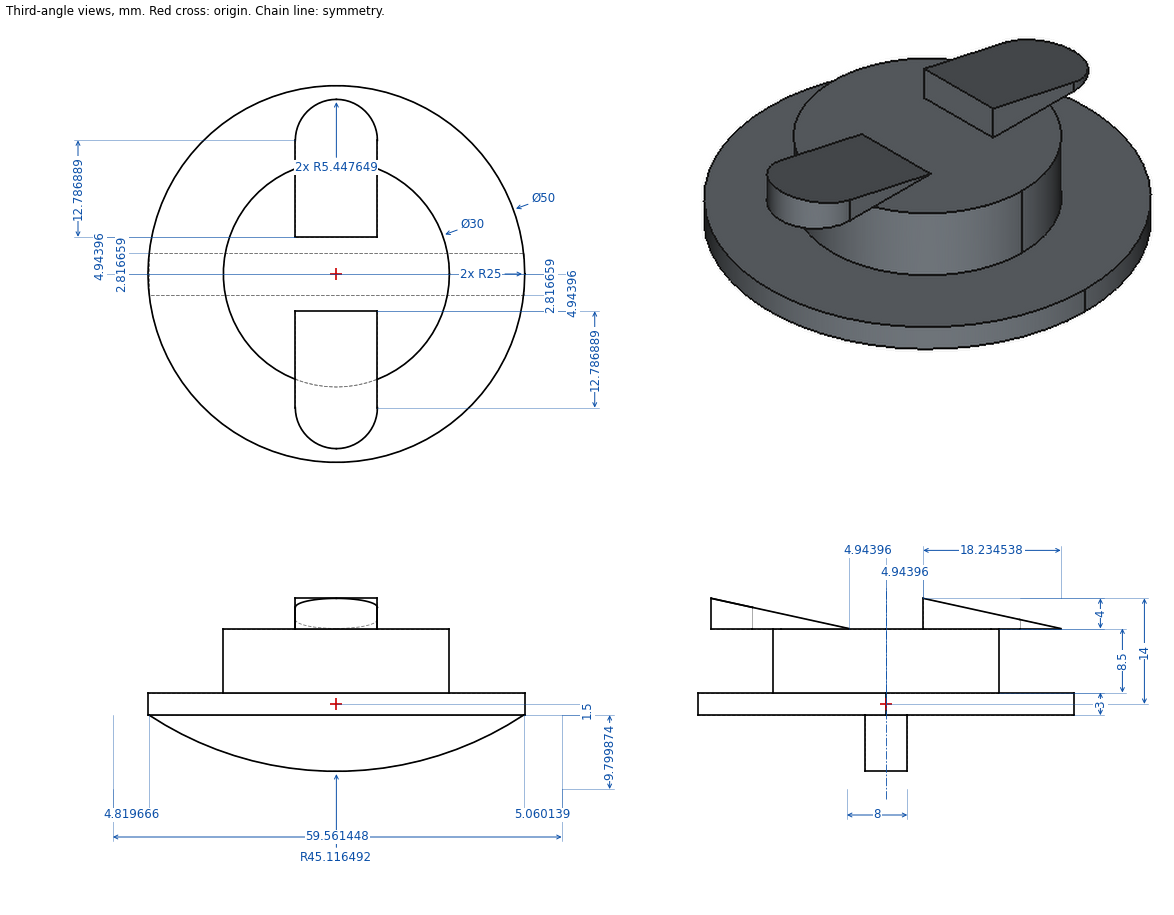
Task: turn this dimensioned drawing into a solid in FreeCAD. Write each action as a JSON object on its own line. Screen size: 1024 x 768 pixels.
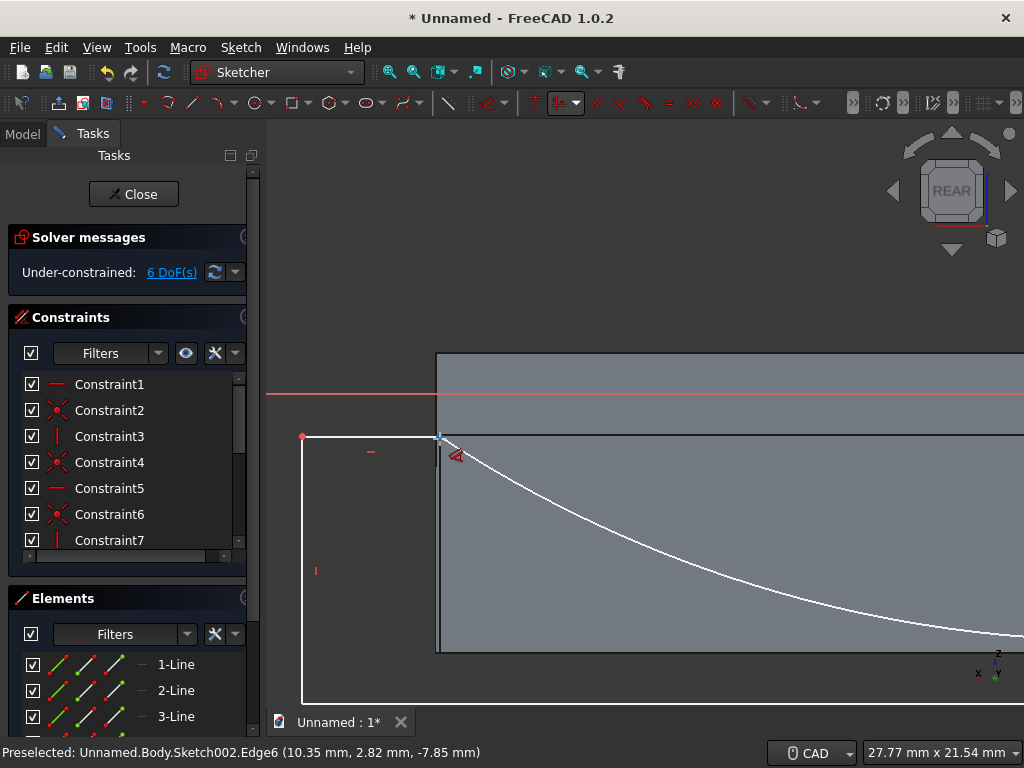
{"action": "left_click", "coordinate": [440, 437]}
{"action": "left_click", "coordinate": [406, 415]}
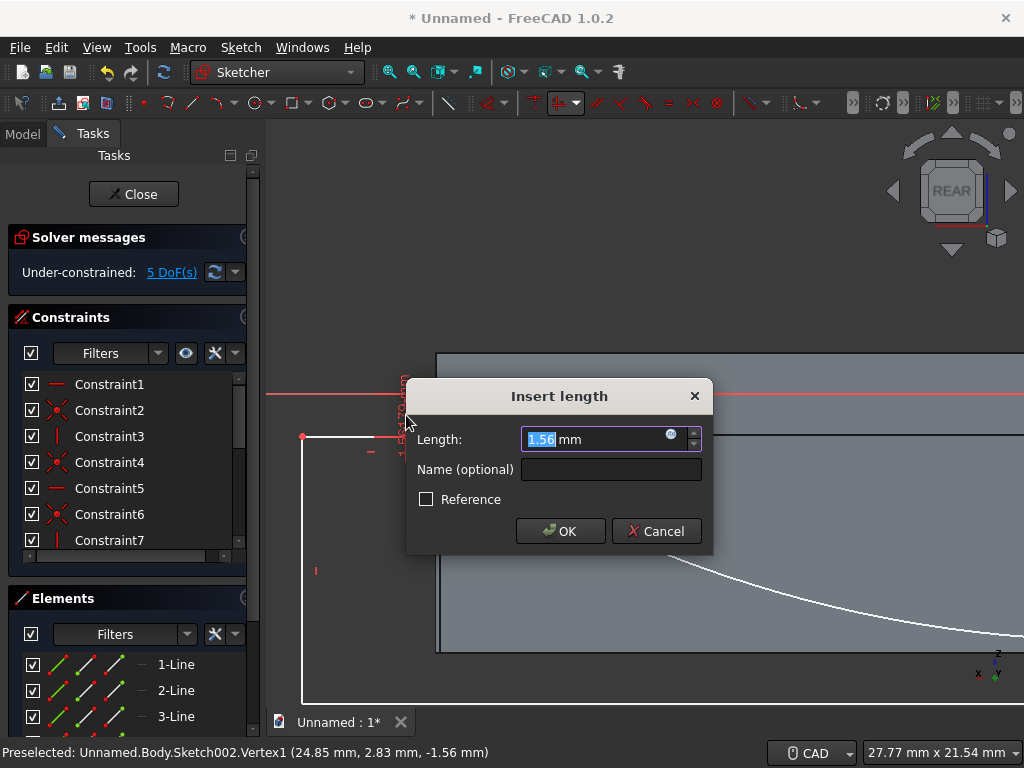
{"action": "type", "text": "1.5"}
{"action": "key", "text": "Return"}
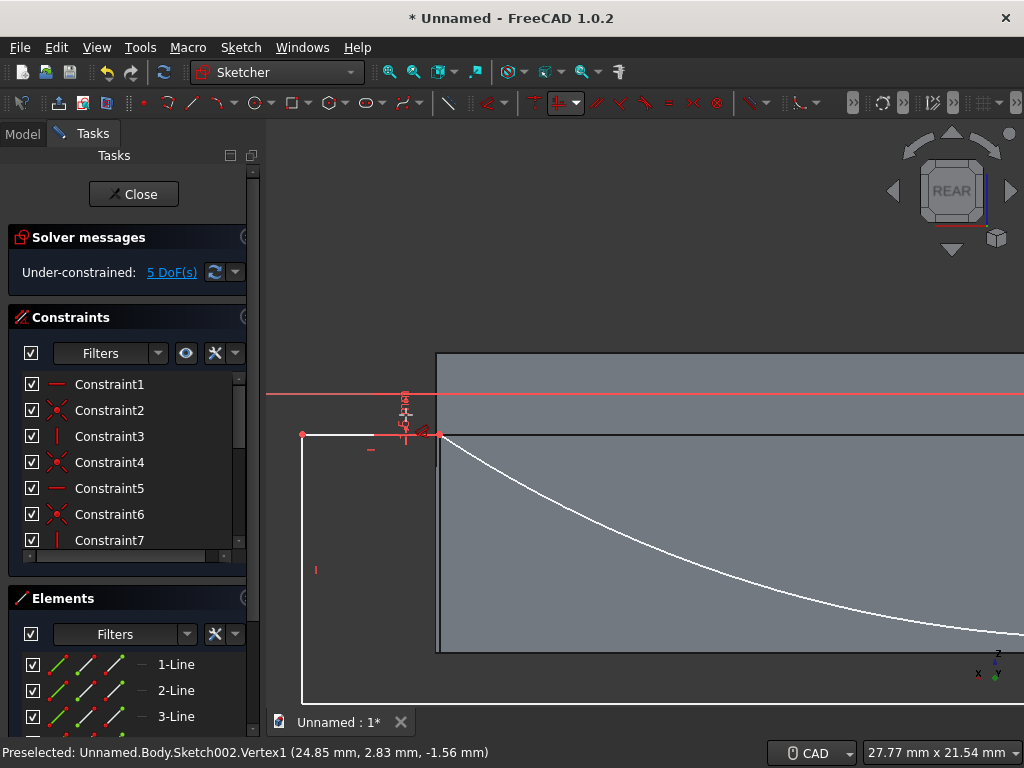
{"action": "scroll", "coordinate": [400, 369], "scroll_direction": "down", "scroll_amount": 7}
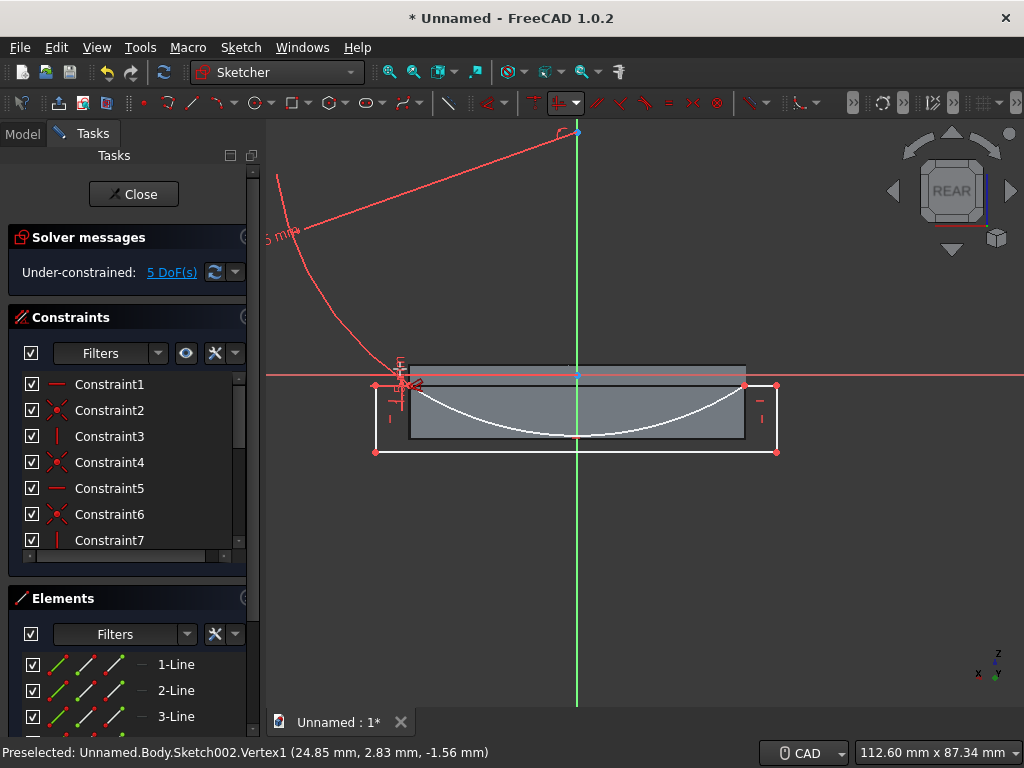
{"action": "scroll", "coordinate": [777, 386], "scroll_direction": "up", "scroll_amount": 7}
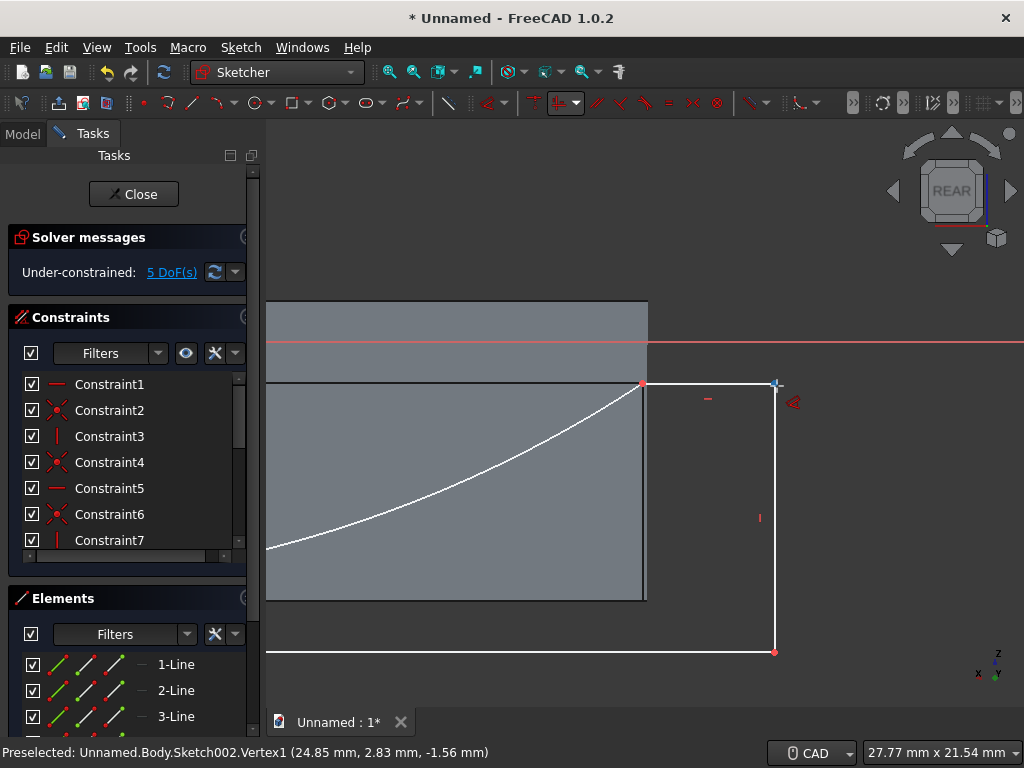
{"action": "left_click", "coordinate": [775, 384]}
{"action": "left_click", "coordinate": [809, 363]}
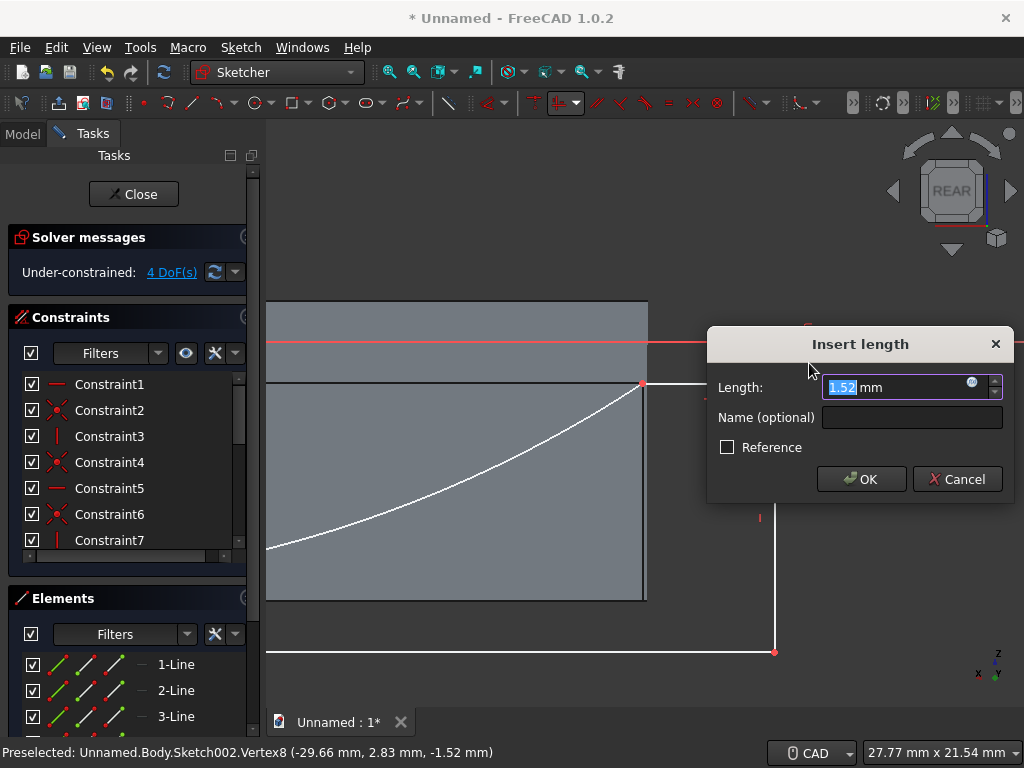
{"action": "type", "text": "1.5"}
{"action": "key", "text": "Return"}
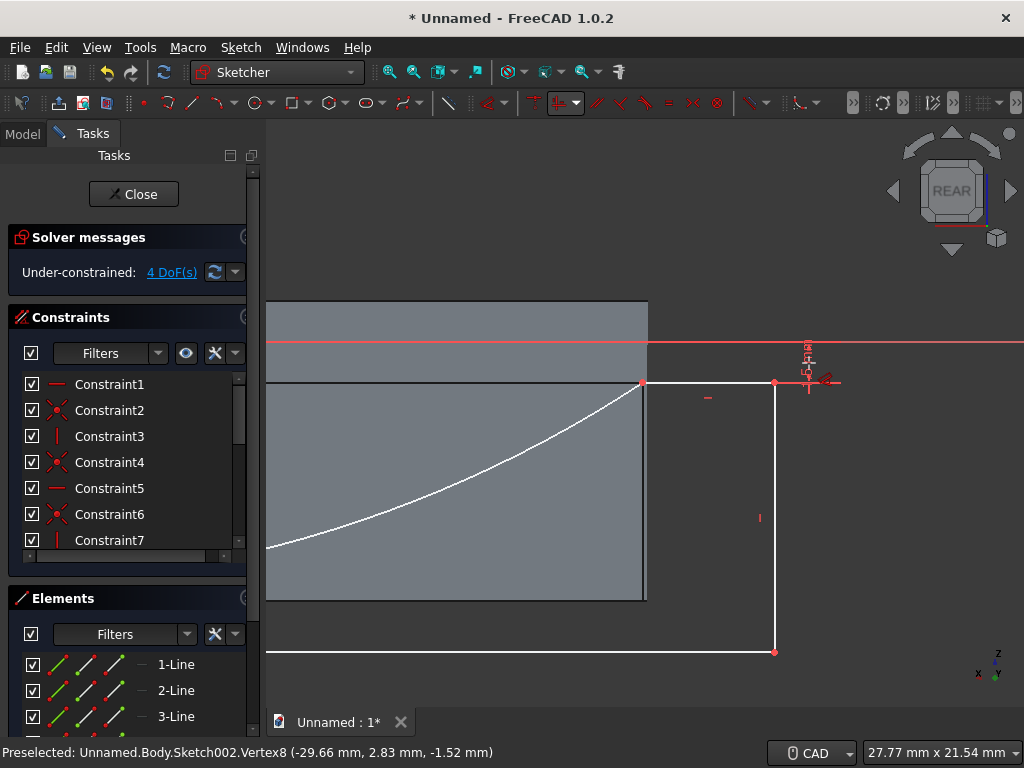
{"action": "scroll", "coordinate": [778, 386], "scroll_direction": "down", "scroll_amount": 7}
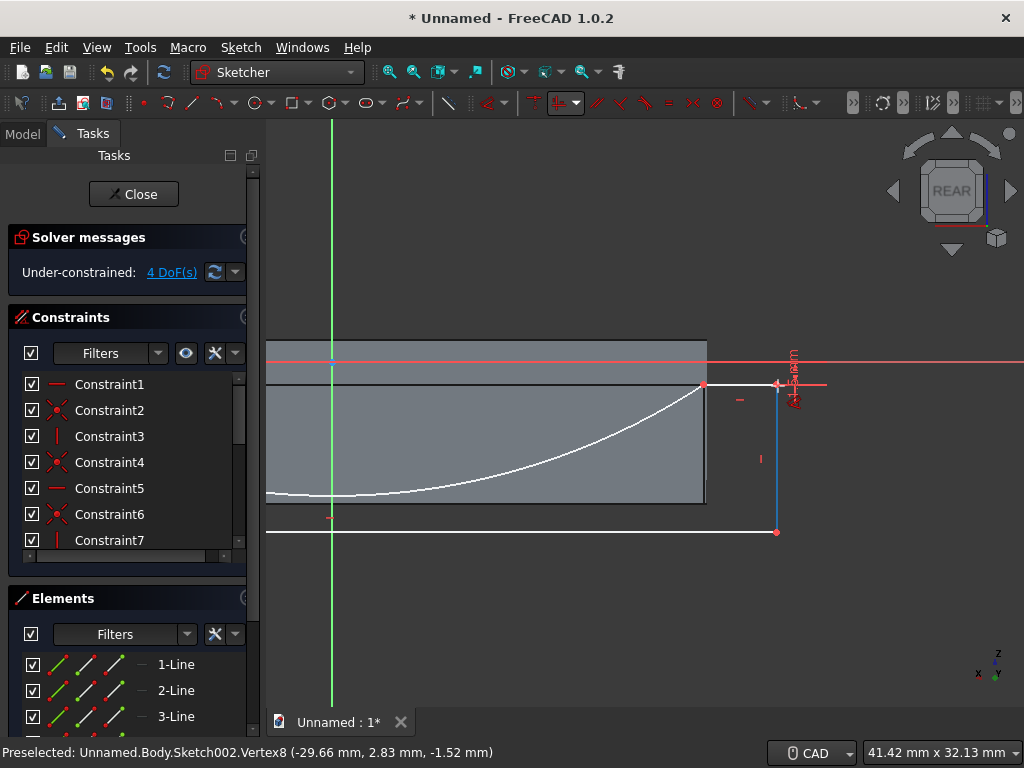
{"action": "scroll", "coordinate": [401, 386], "scroll_direction": "up", "scroll_amount": 2}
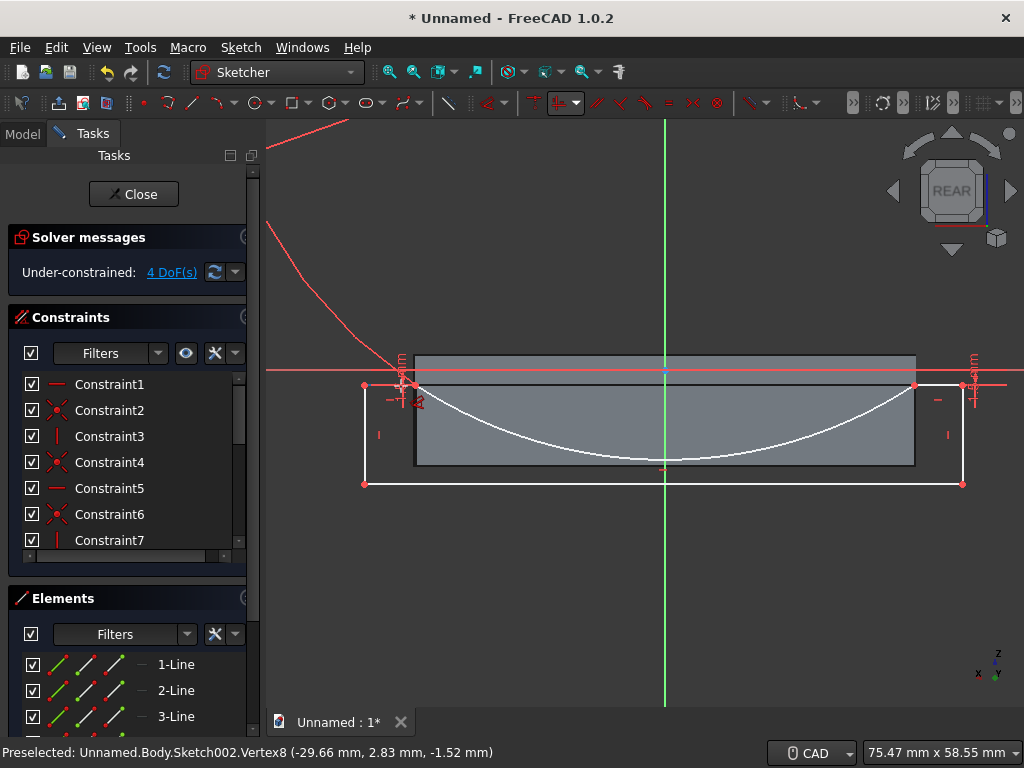
{"action": "left_click", "coordinate": [400, 385]}
{"action": "left_click", "coordinate": [390, 351]}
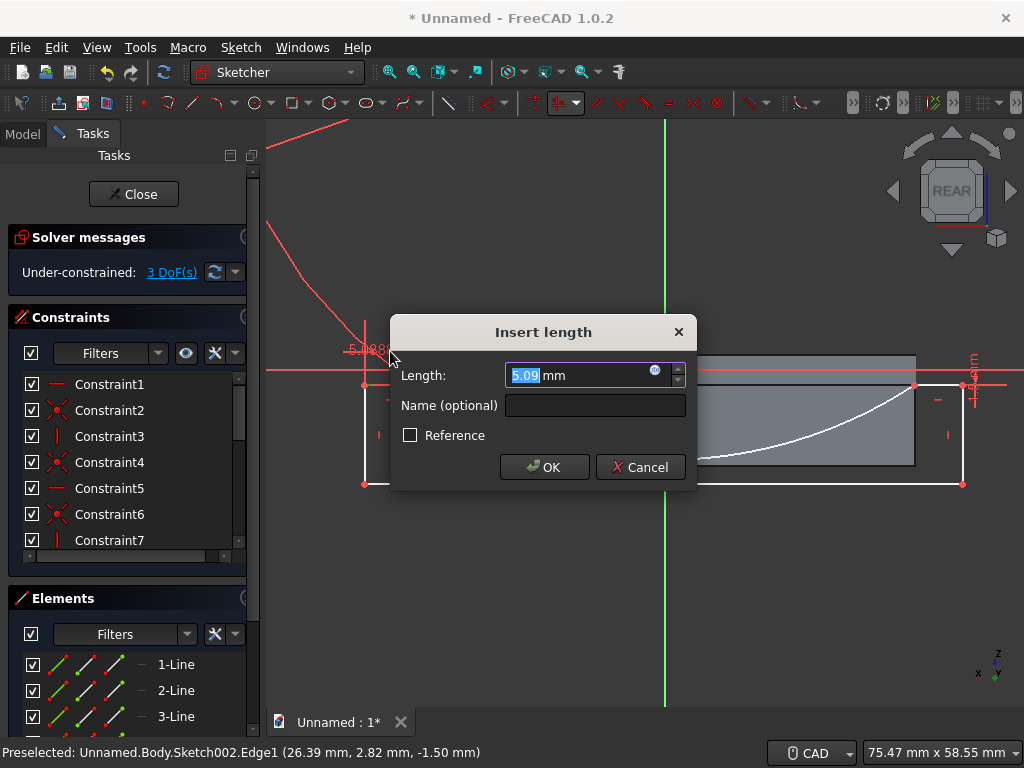
{"action": "type", "text": "5.060139"}
{"action": "key", "text": "Return"}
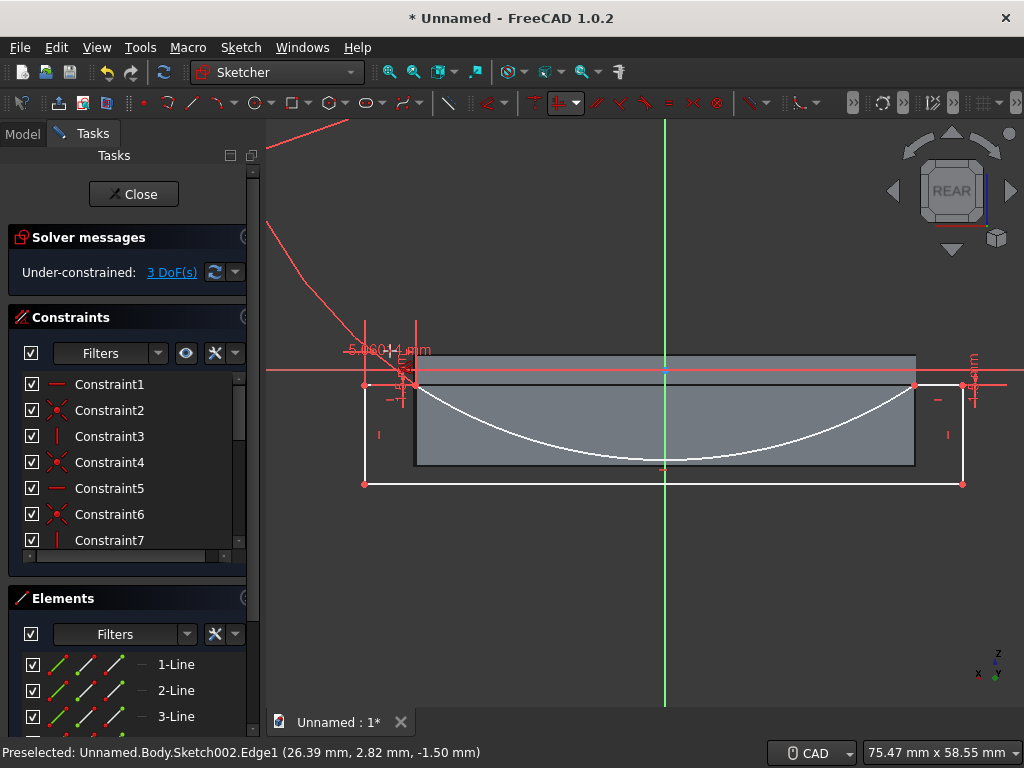
{"action": "left_click", "coordinate": [365, 415]}
{"action": "left_click", "coordinate": [331, 435]}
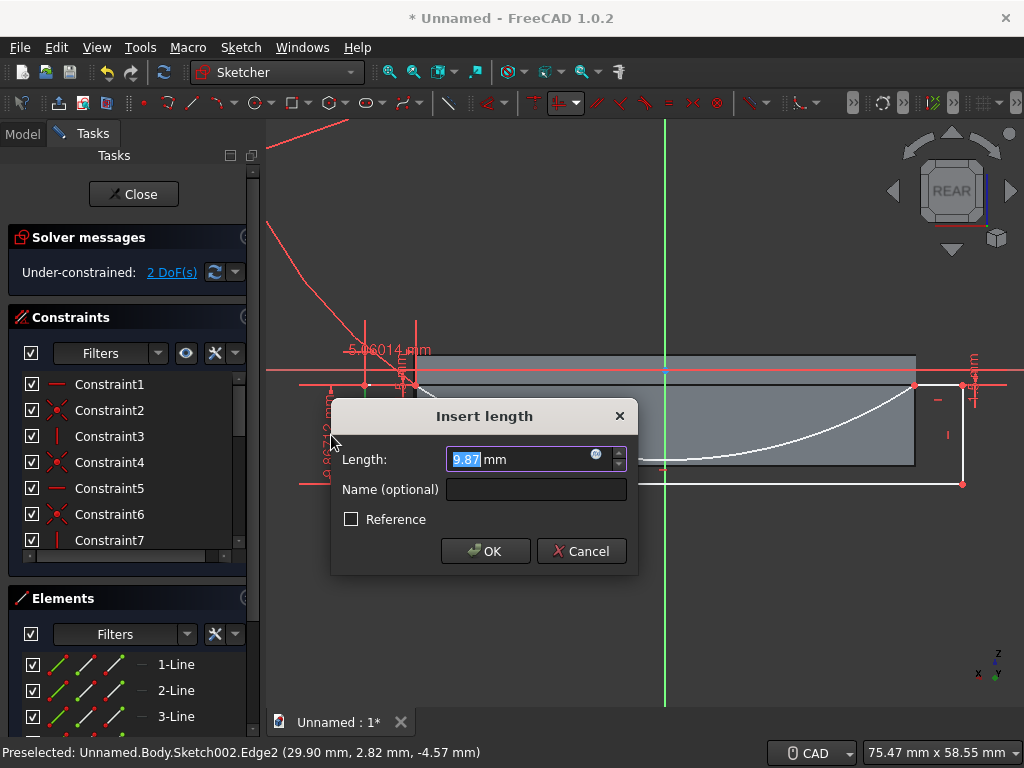
{"action": "type", "text": "9.799874"}
{"action": "key", "text": "Return"}